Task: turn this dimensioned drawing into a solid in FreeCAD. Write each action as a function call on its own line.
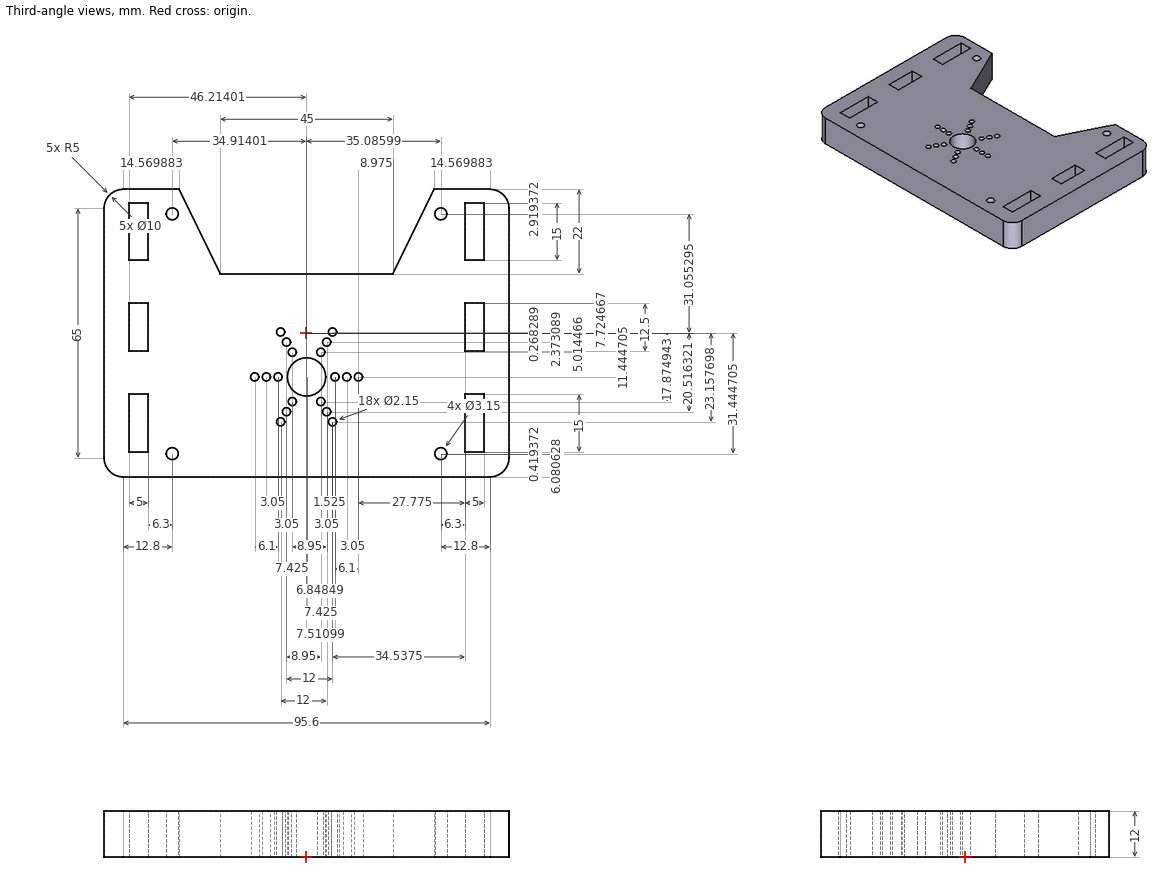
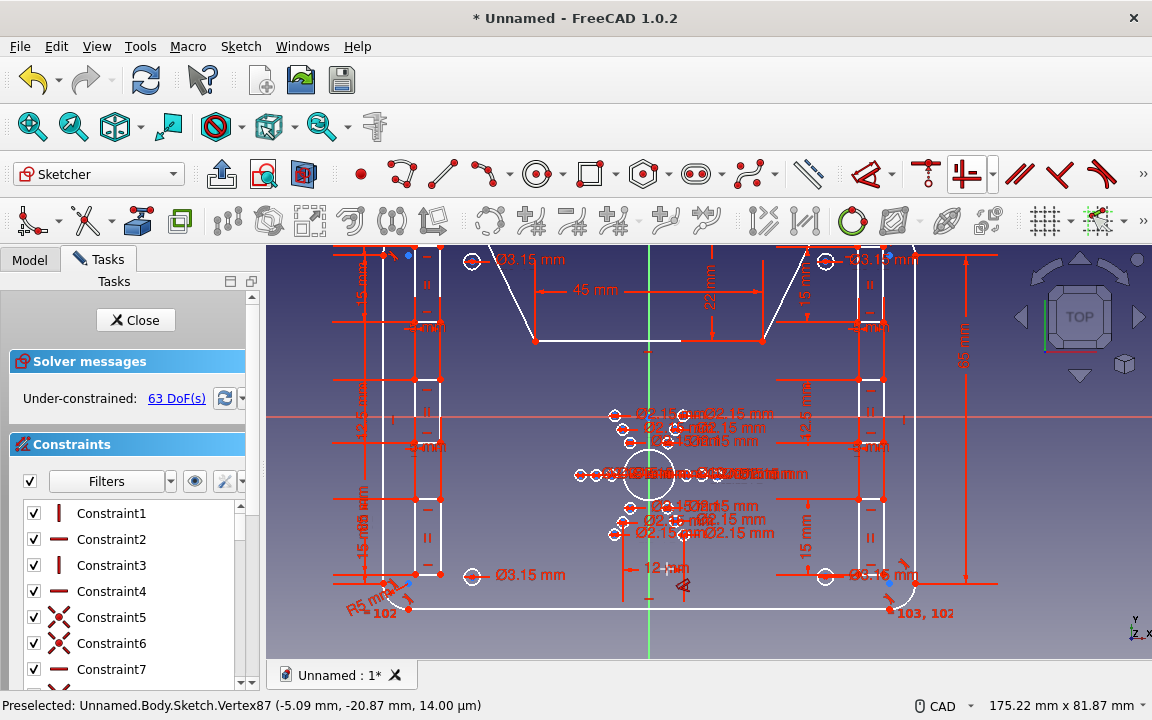
click(675, 521)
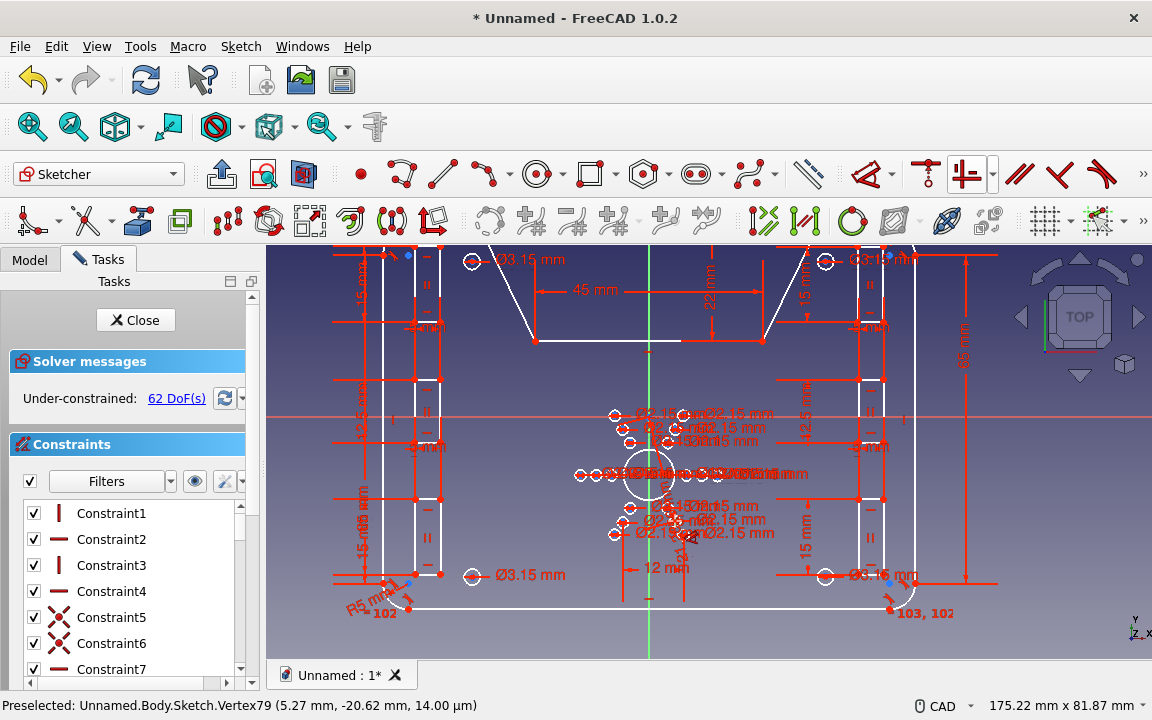
click(615, 535)
click(631, 593)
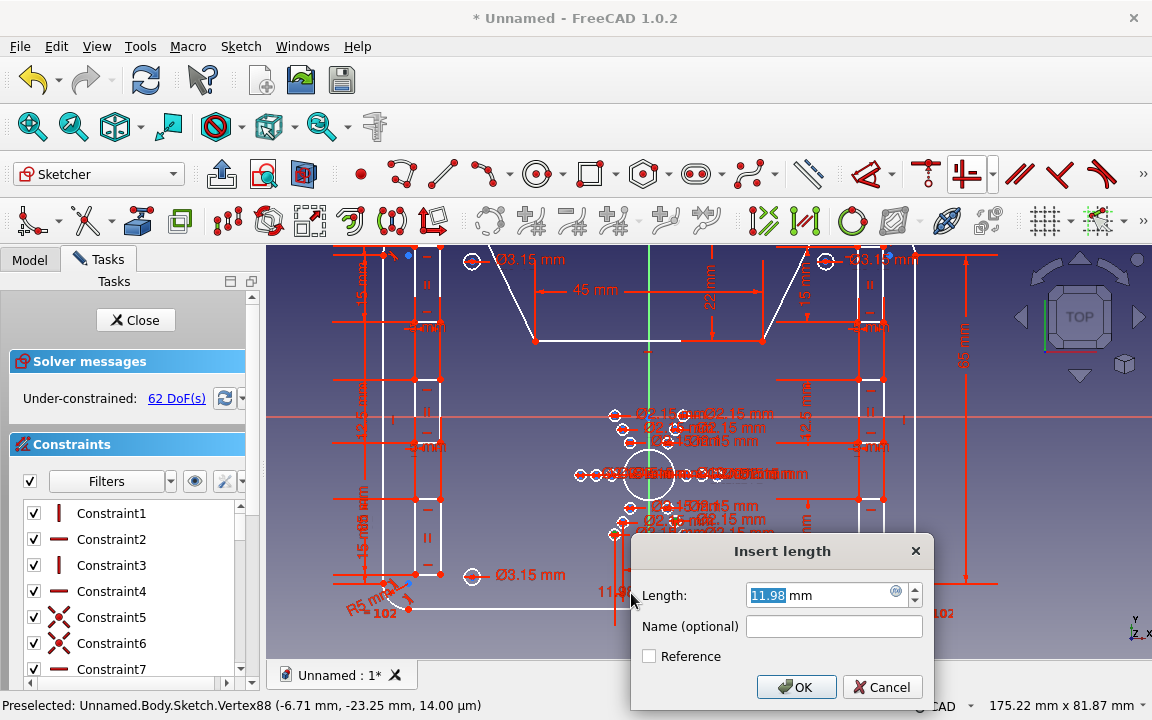
text(12)
key(Return)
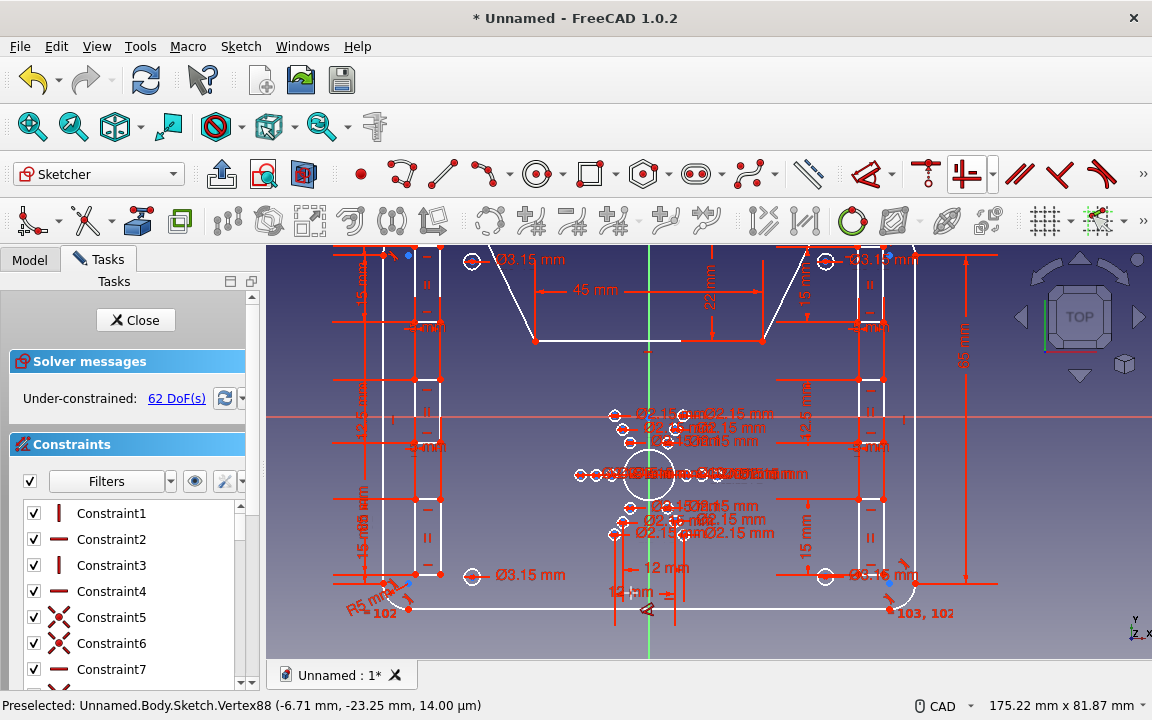
click(675, 430)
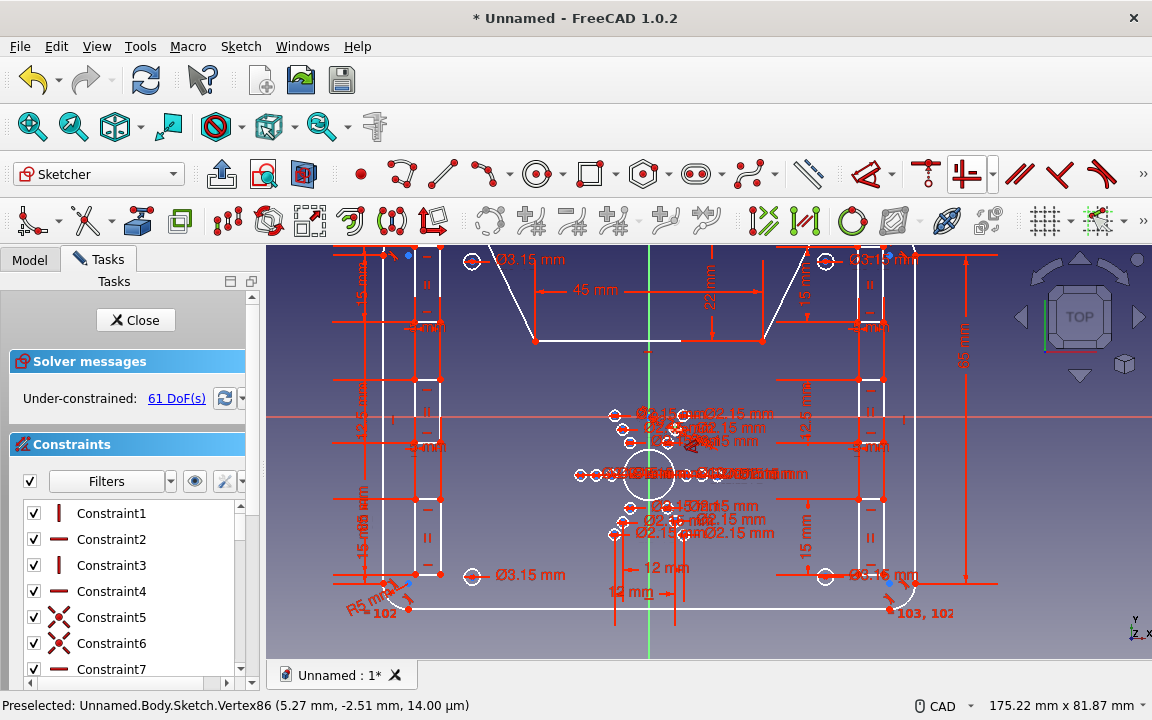
click(615, 416)
click(631, 382)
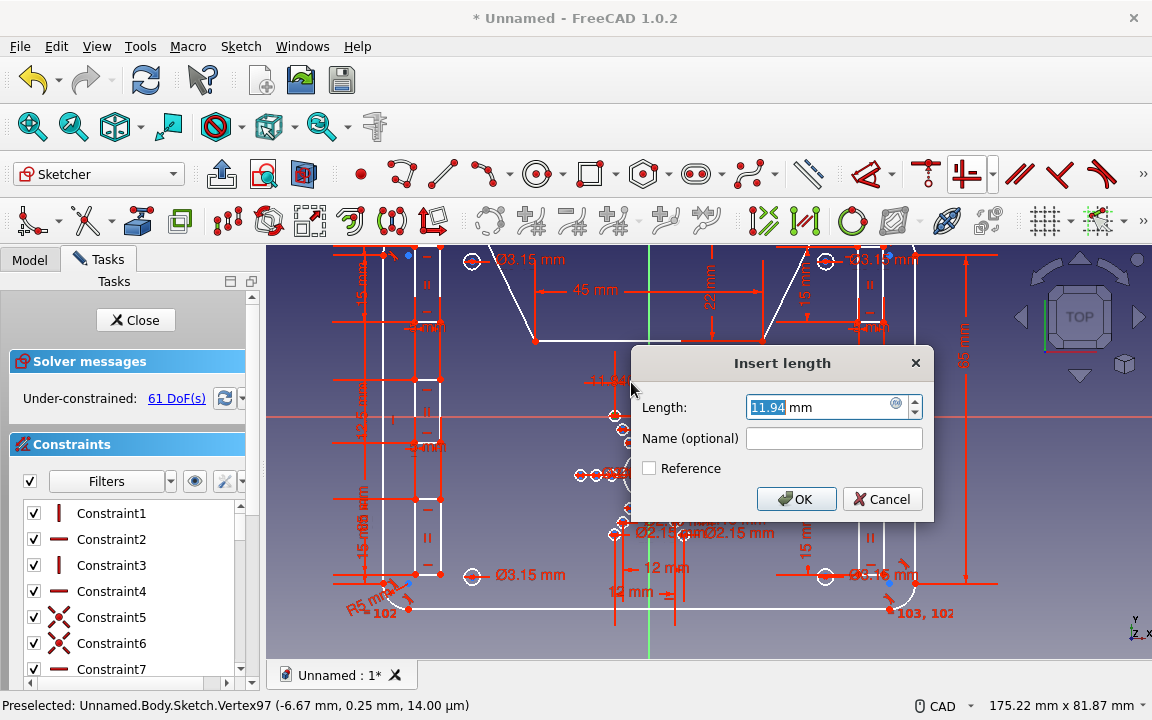
text(12)
key(Return)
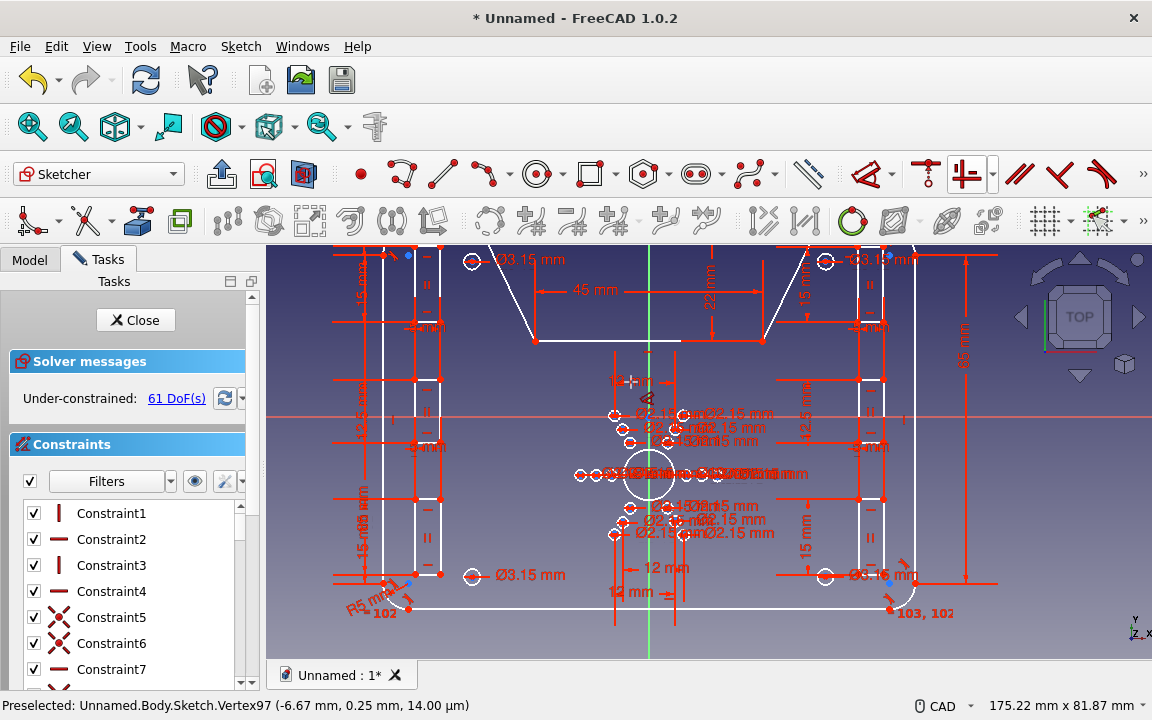
click(553, 609)
click(538, 575)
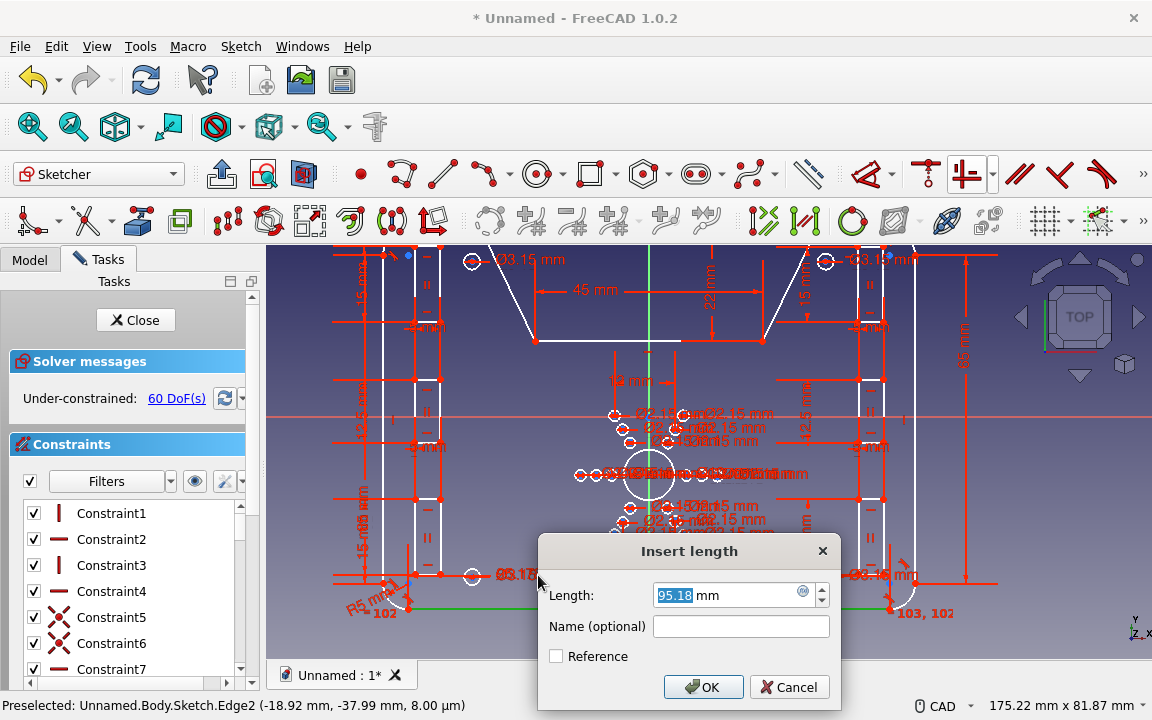
text(95.6)
key(Return)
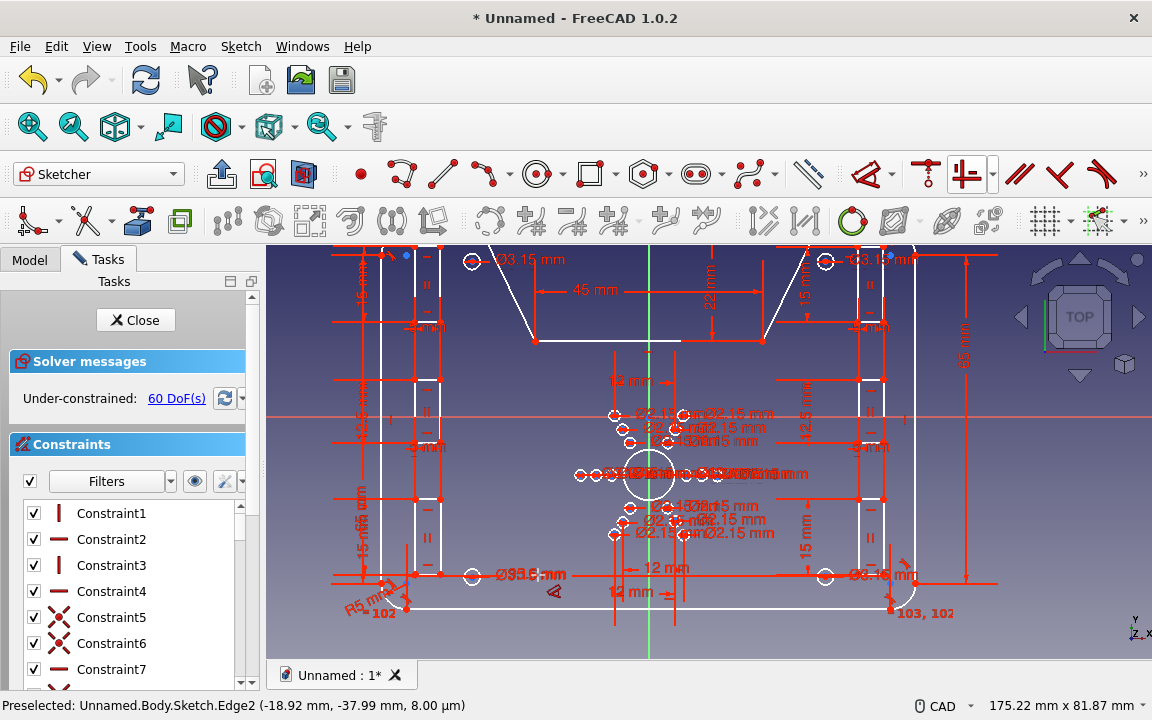
scroll(859, 575, up, 2)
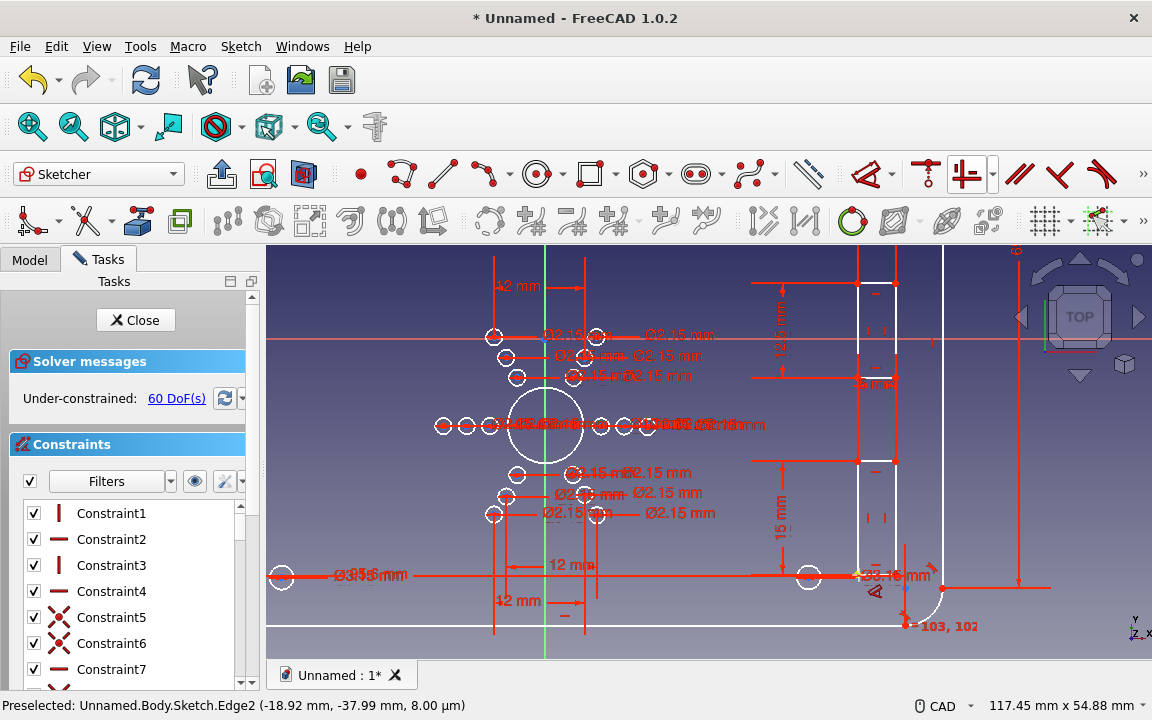
click(858, 575)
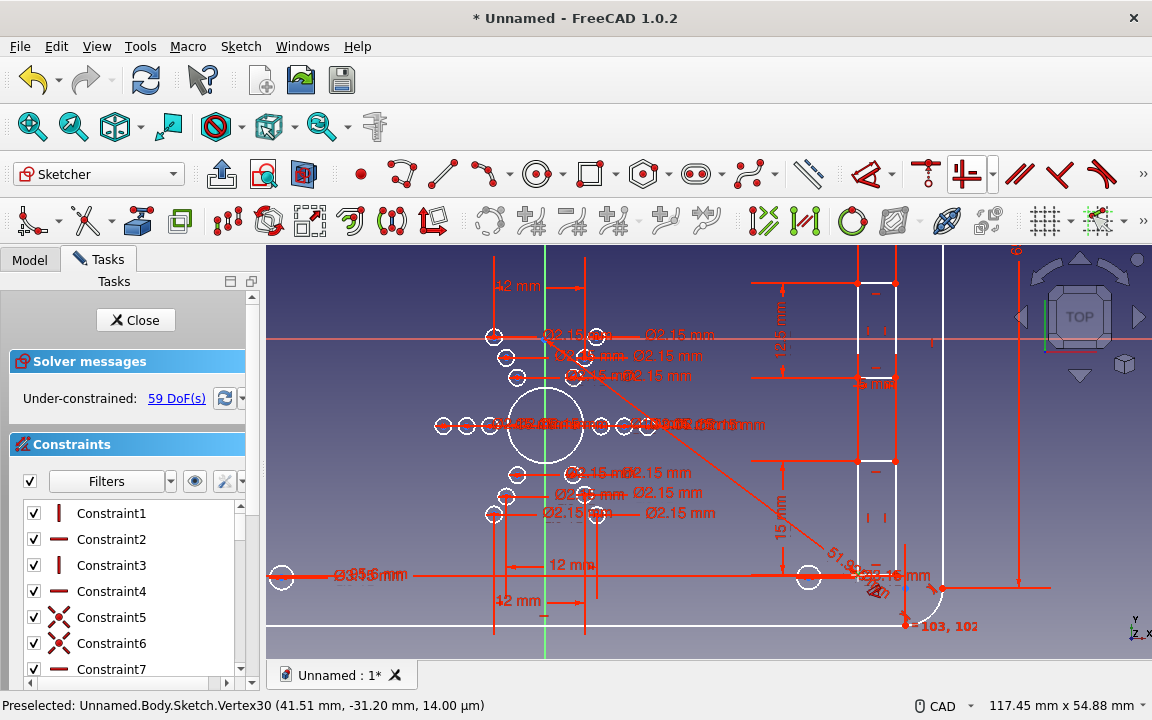
click(809, 578)
click(833, 612)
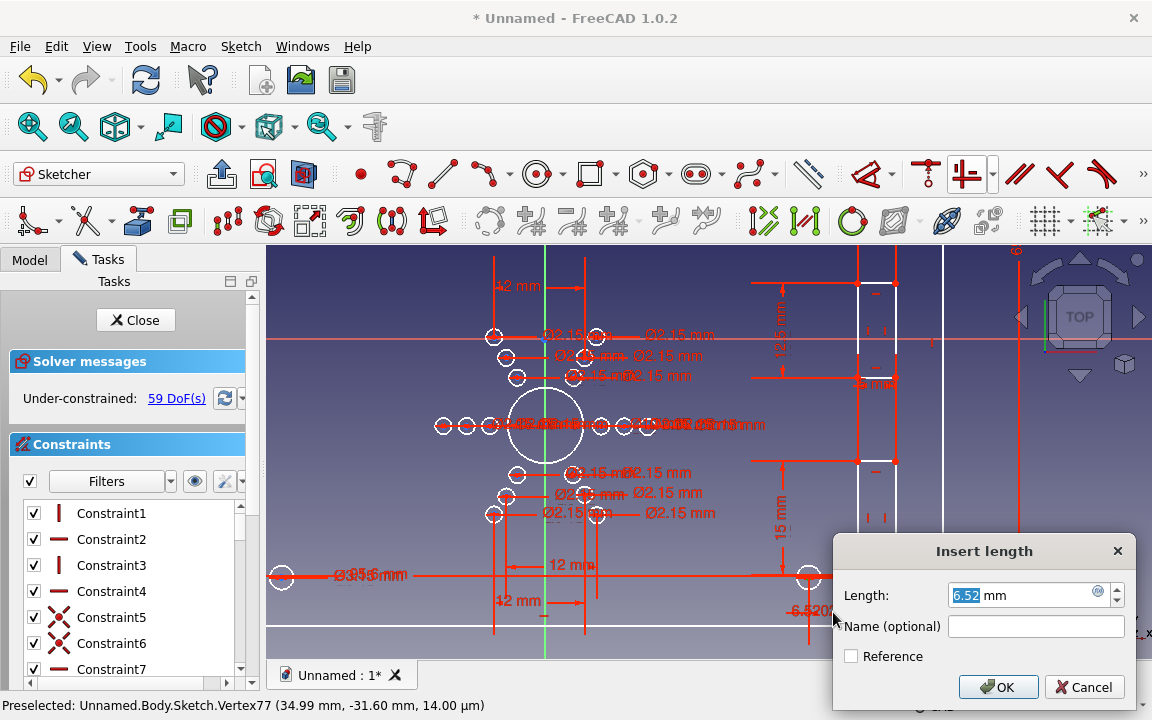
text(6.3)
key(Return)